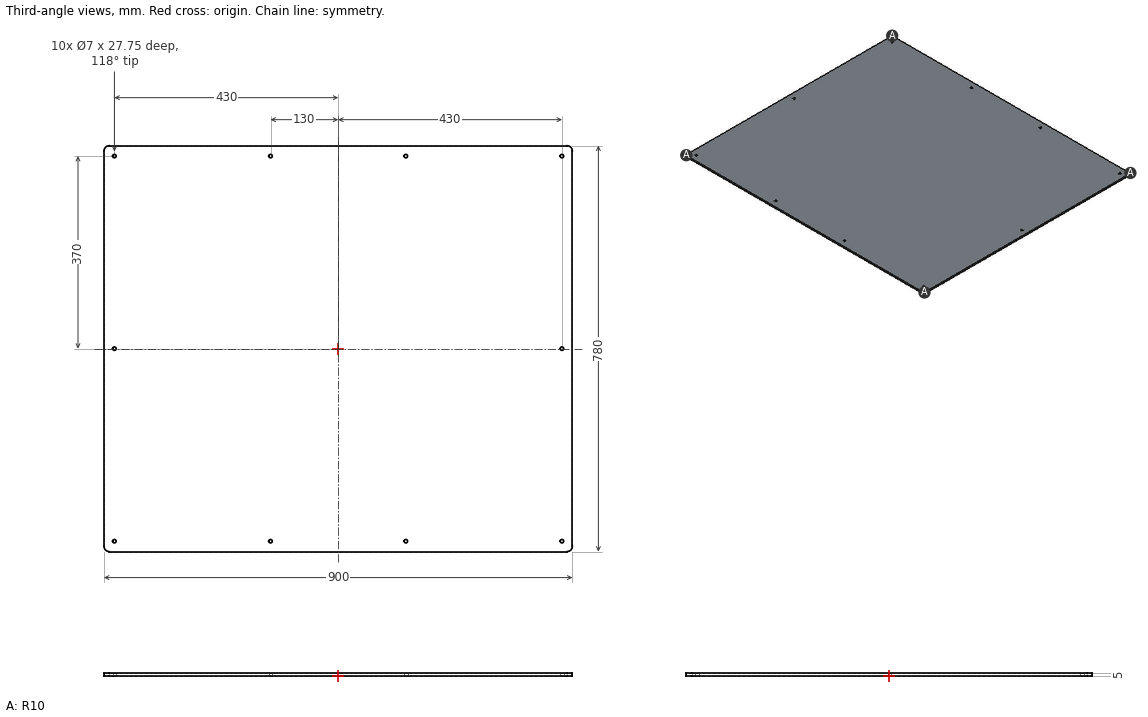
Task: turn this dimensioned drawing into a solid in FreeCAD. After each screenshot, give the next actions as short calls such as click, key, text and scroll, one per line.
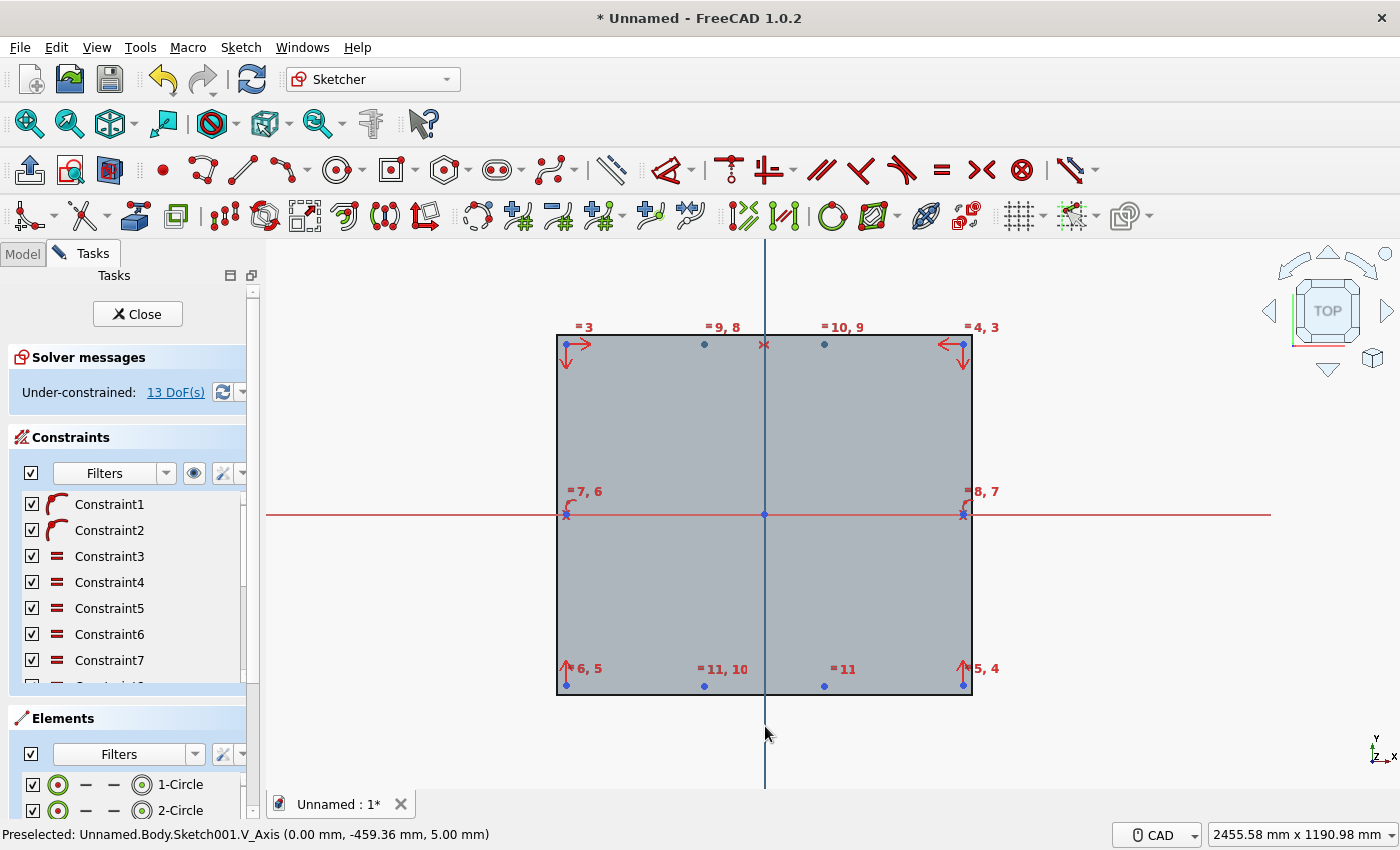
click(982, 170)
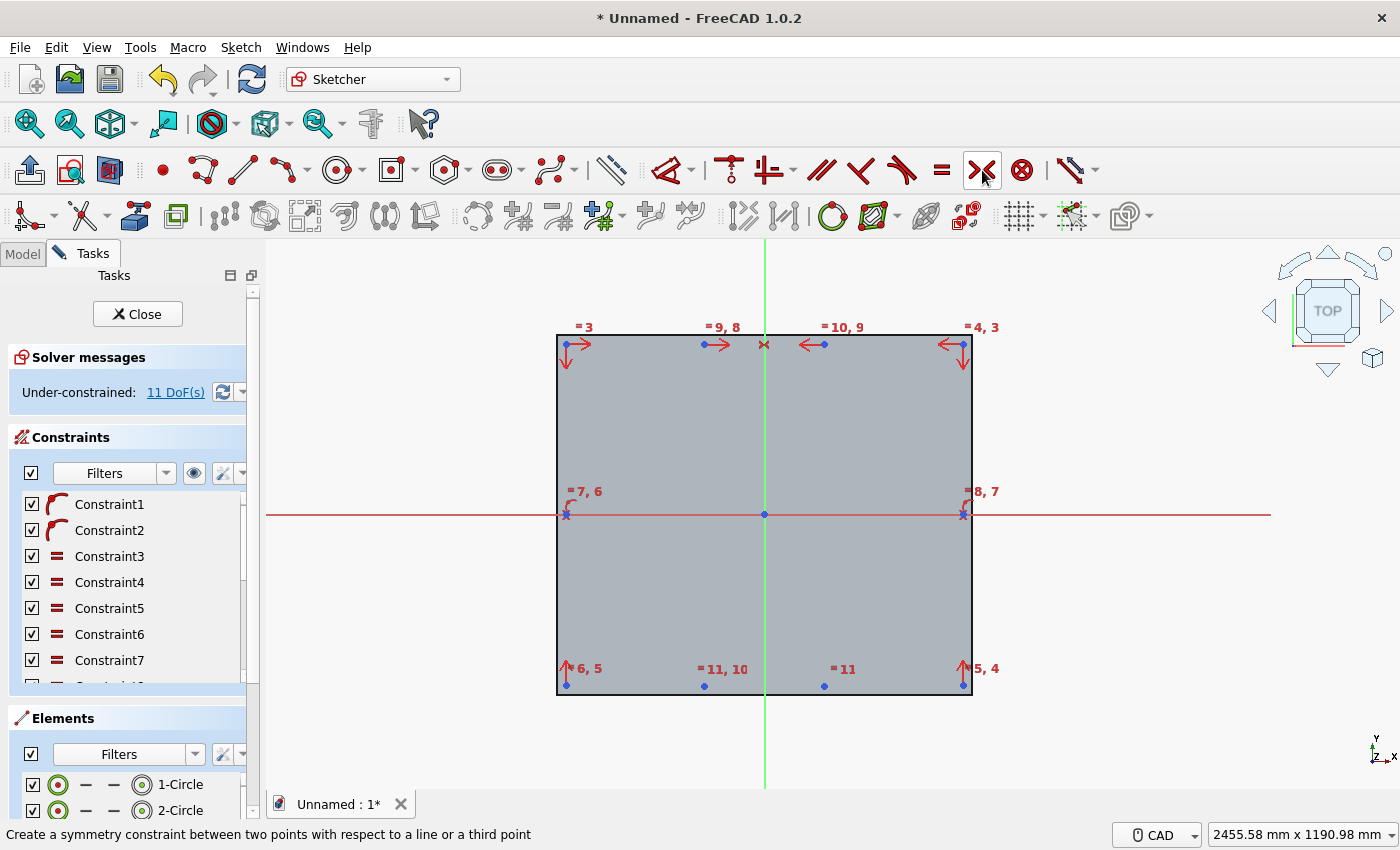
click(705, 345)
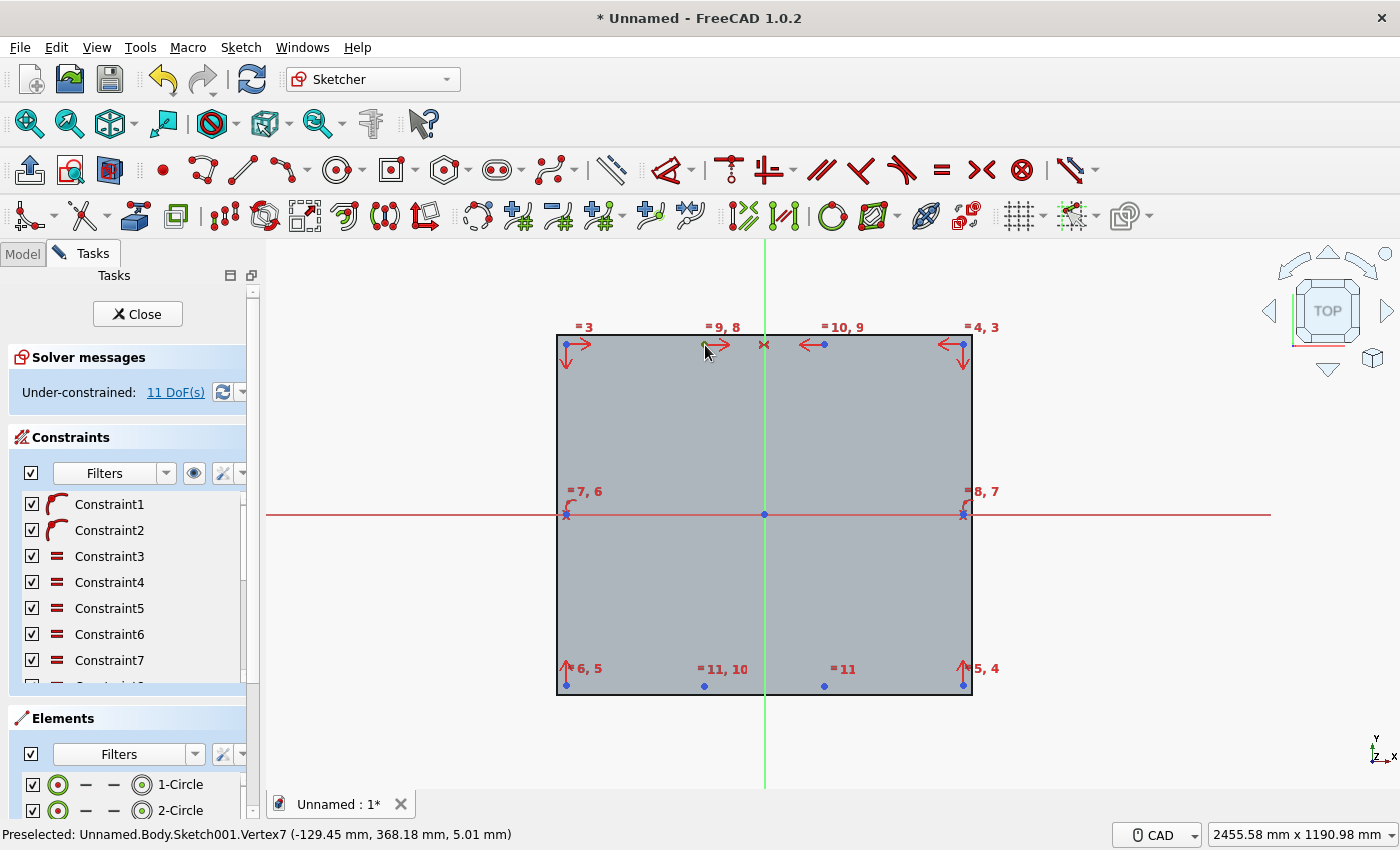
click(704, 687)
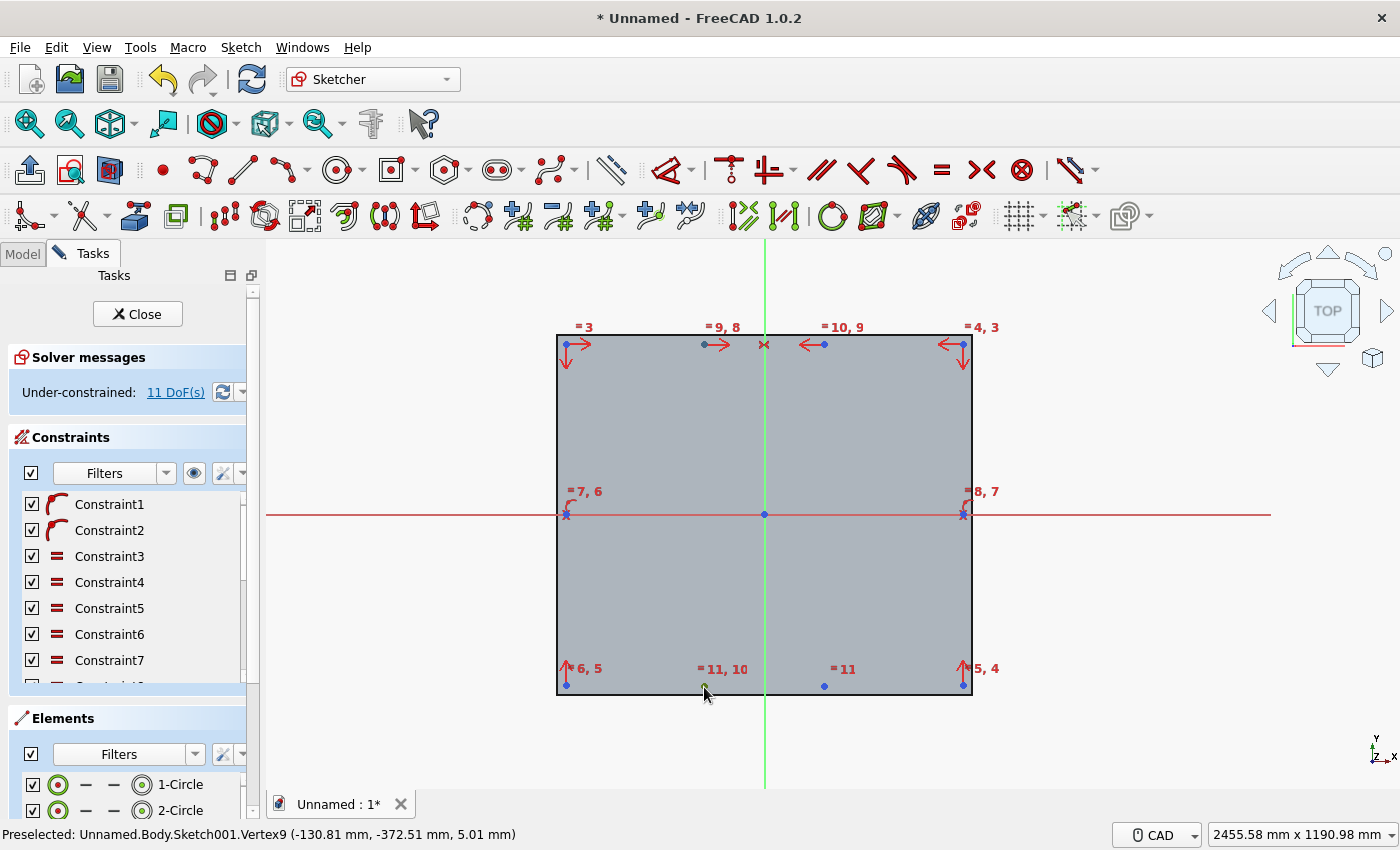
click(361, 515)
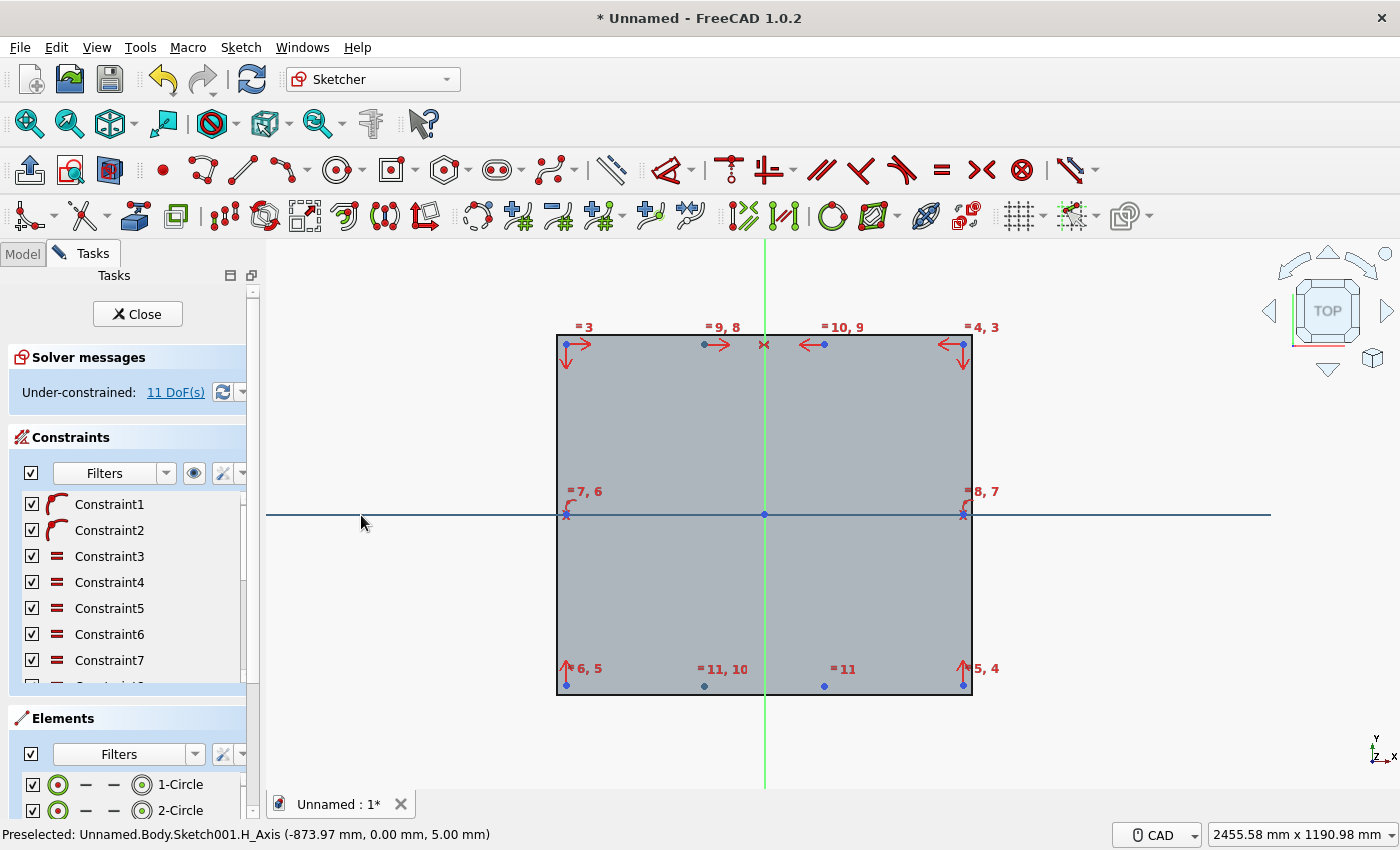
click(982, 170)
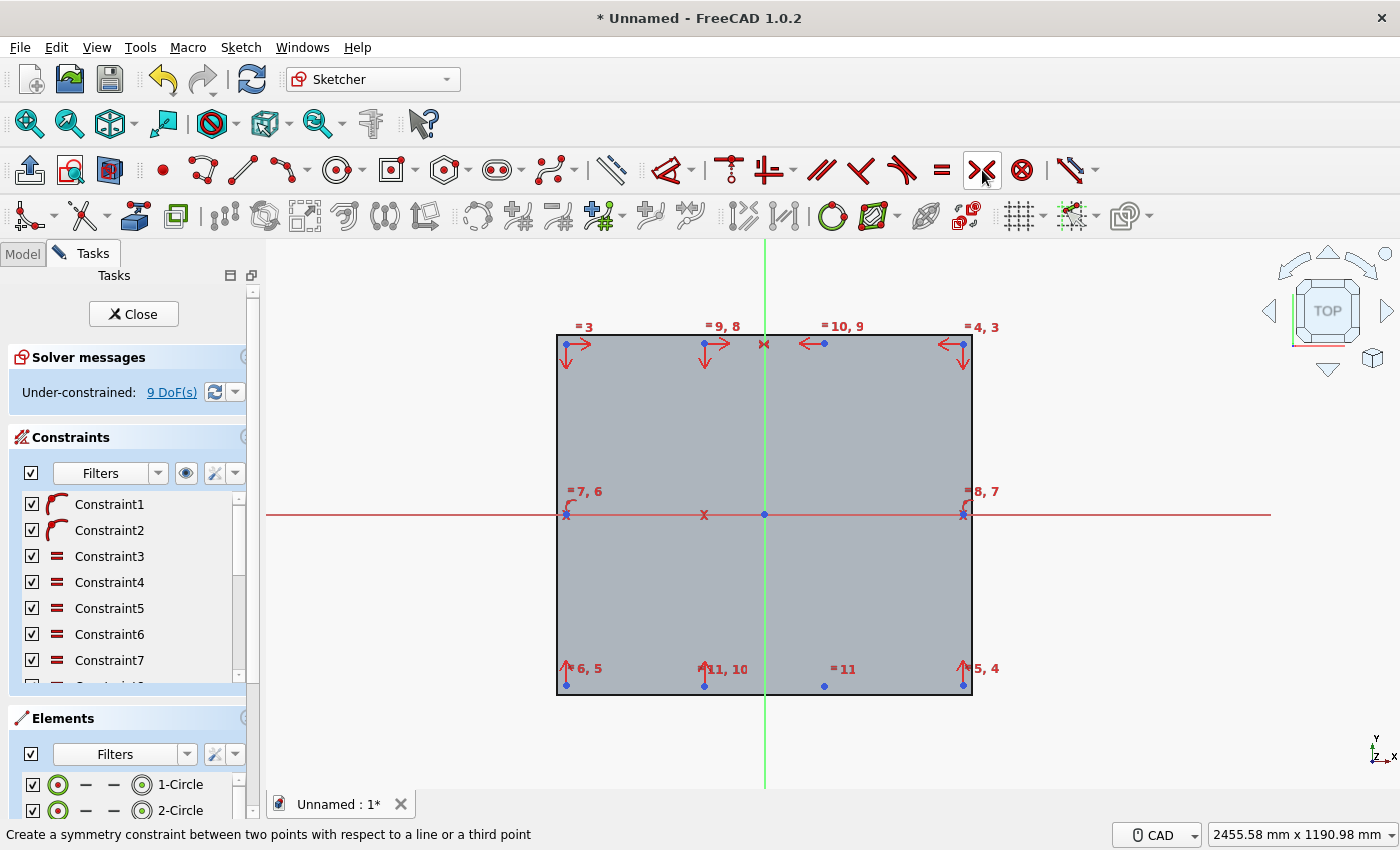
click(824, 344)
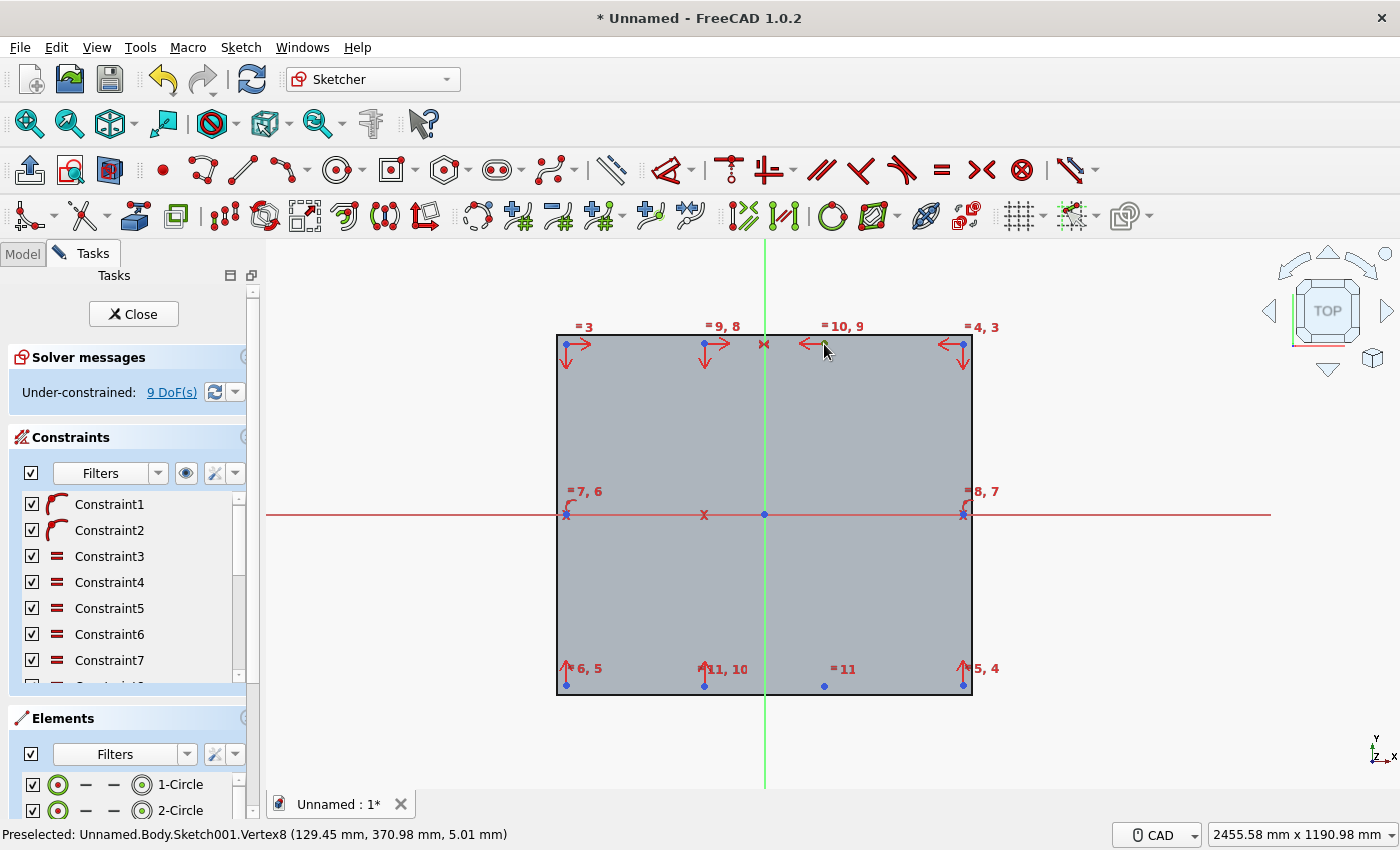
click(824, 687)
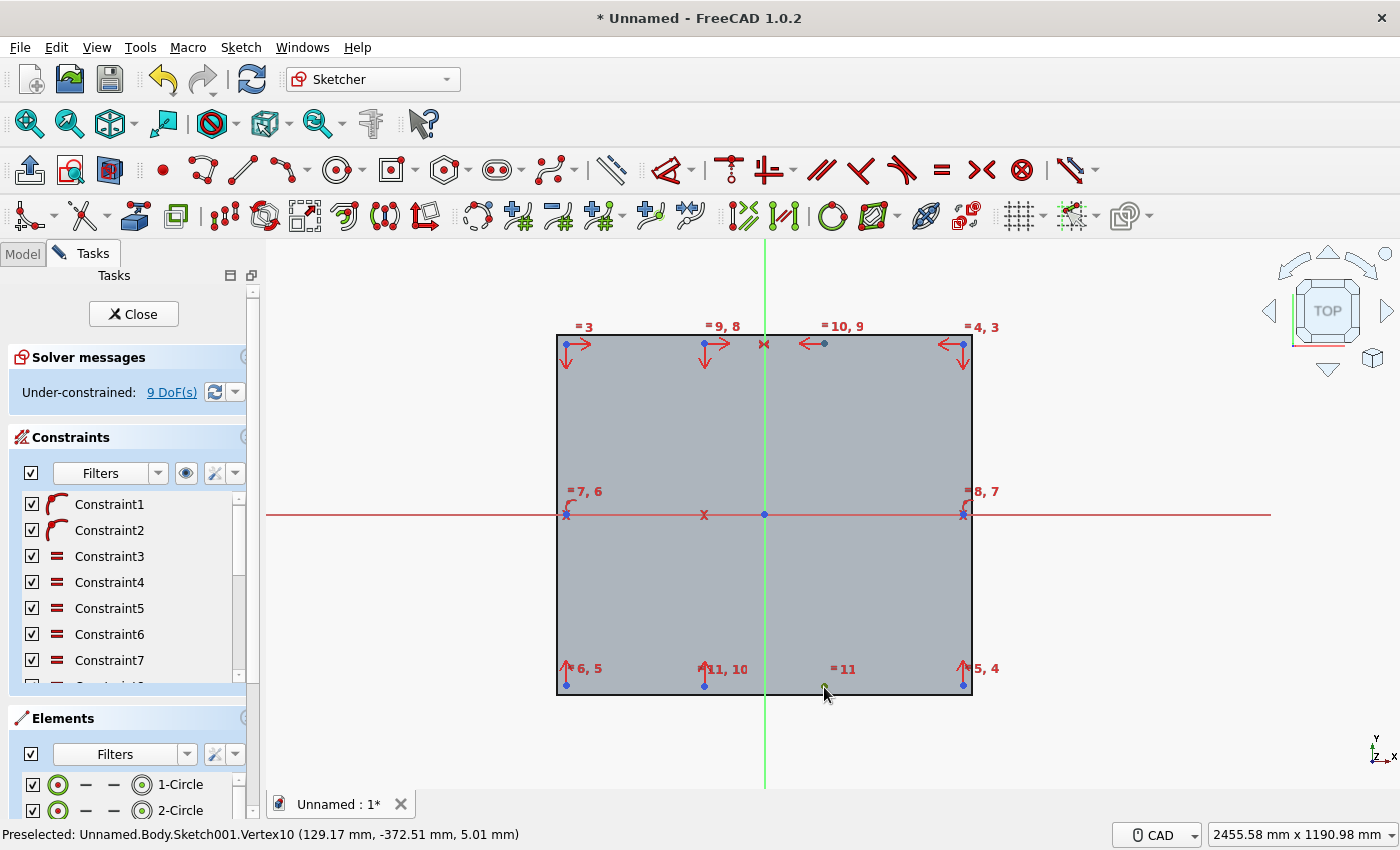
click(361, 515)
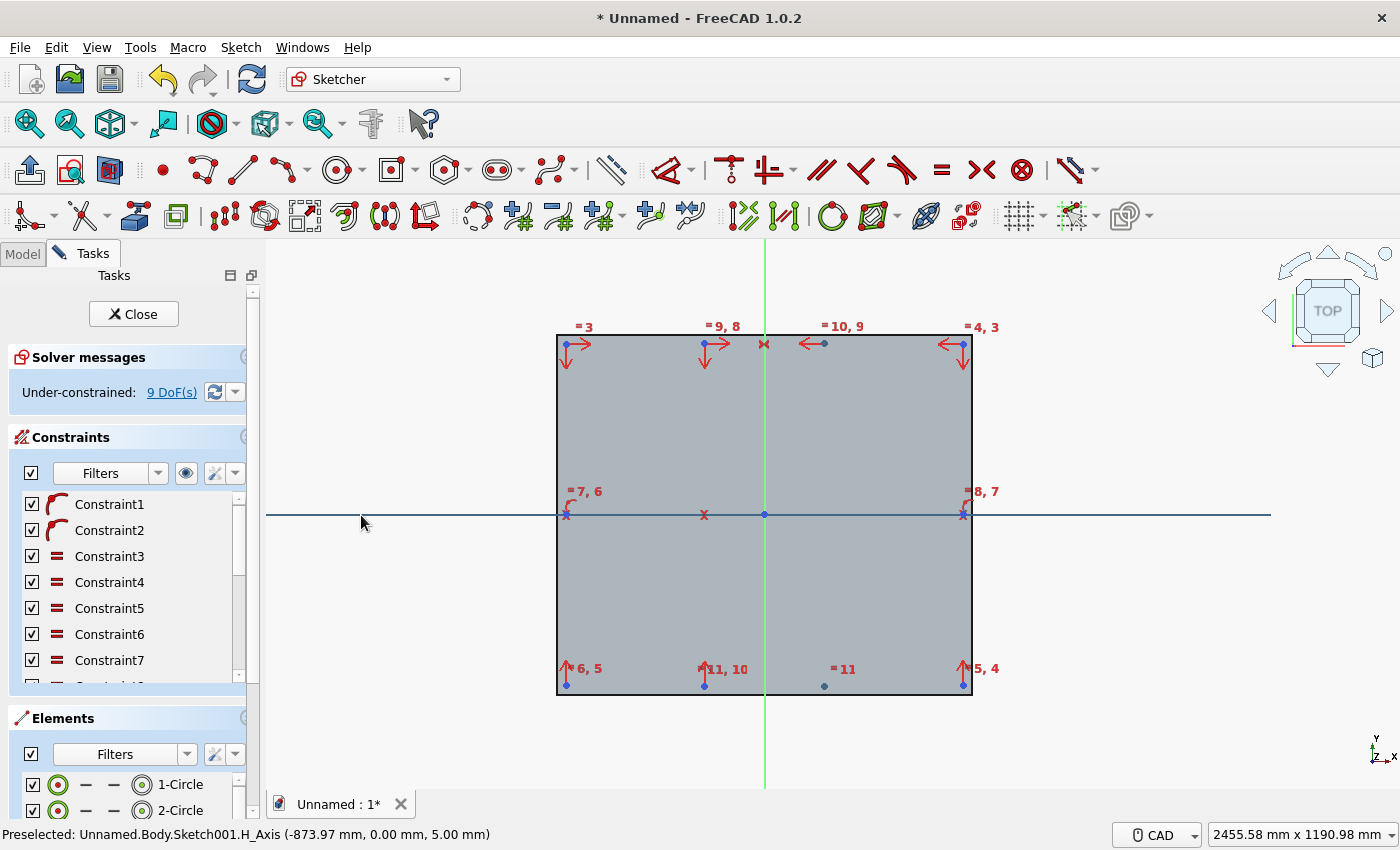
click(982, 170)